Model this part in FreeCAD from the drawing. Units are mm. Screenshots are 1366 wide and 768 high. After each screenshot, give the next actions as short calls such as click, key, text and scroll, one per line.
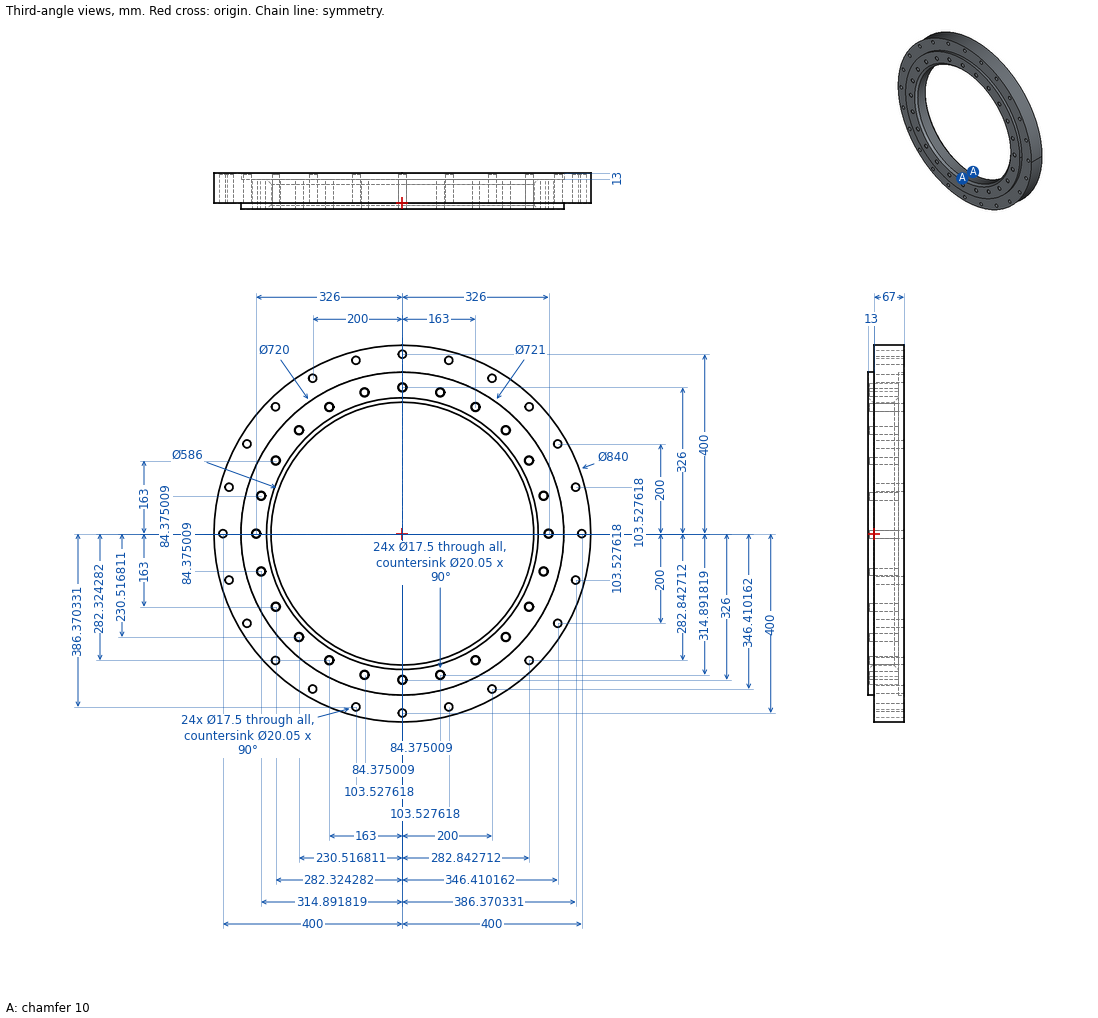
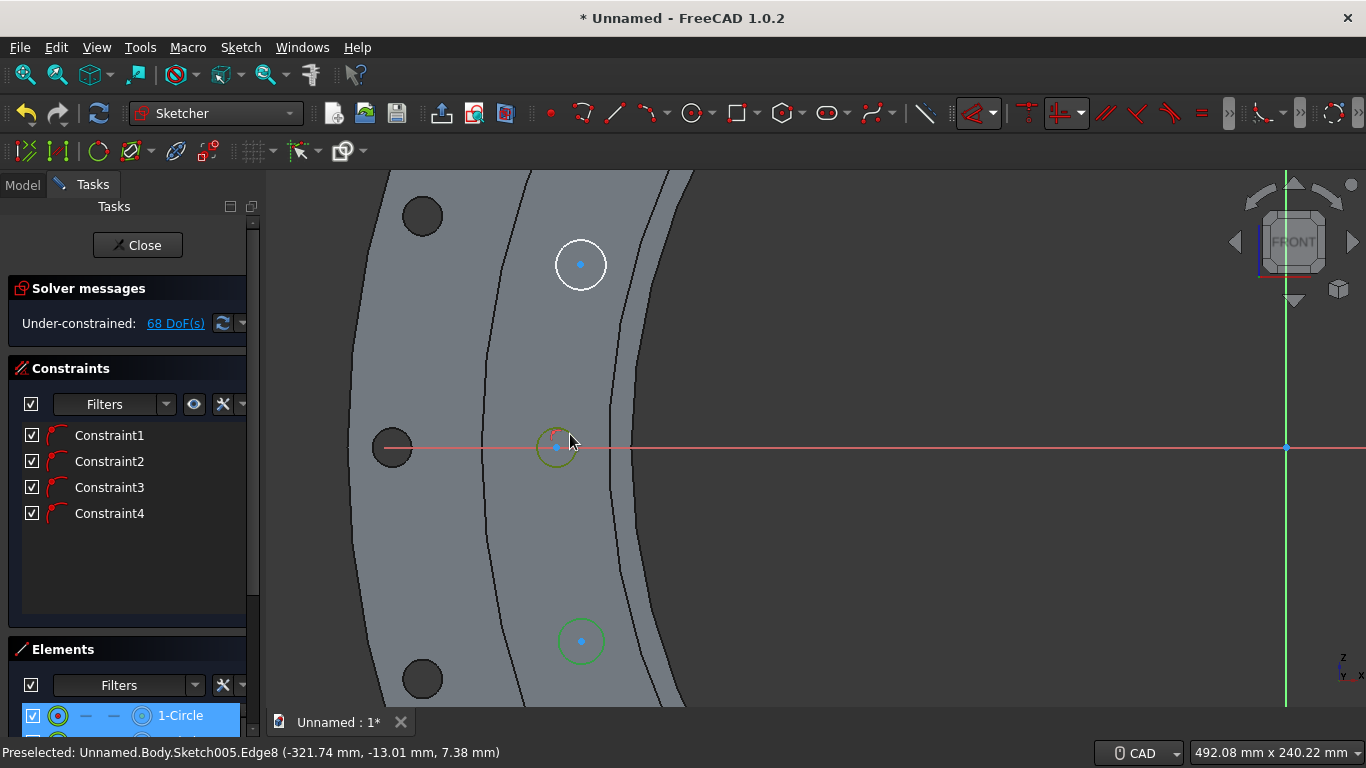
click(598, 247)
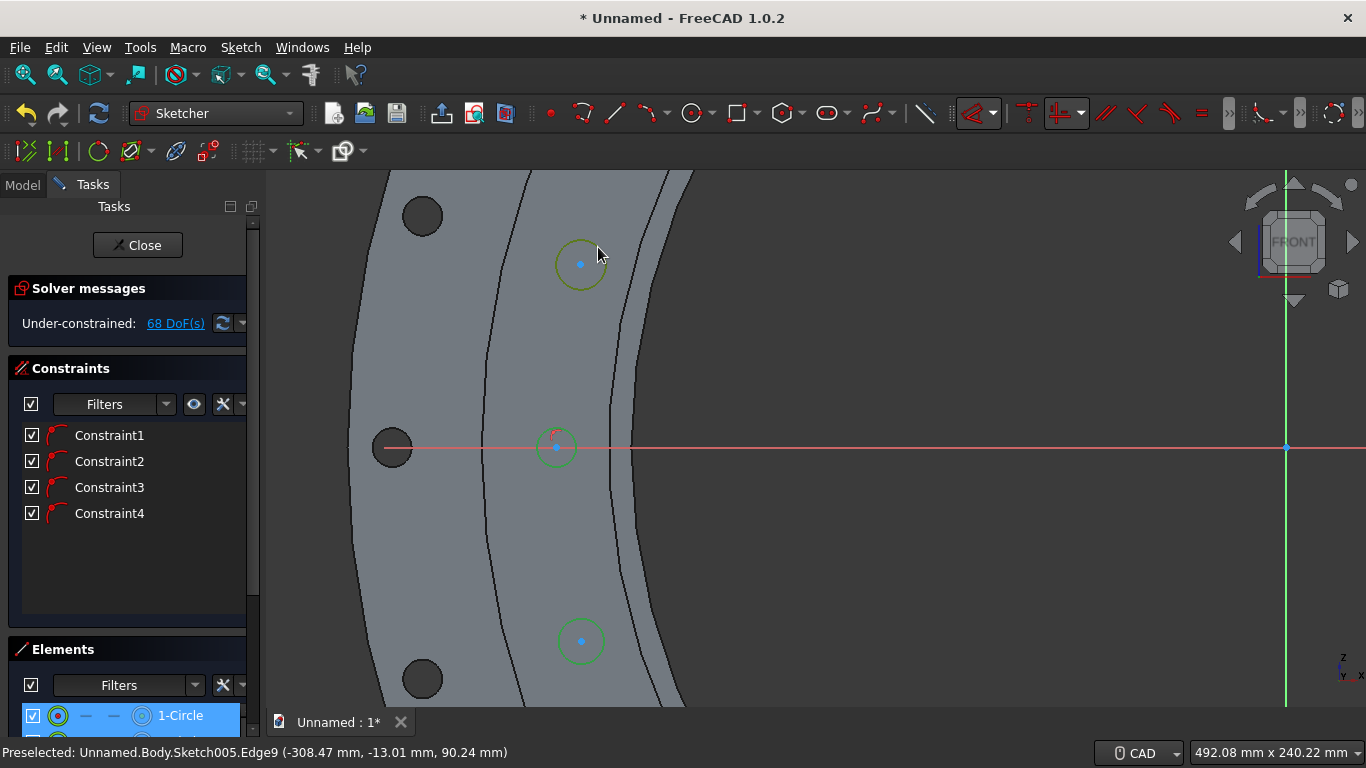
scroll(571, 436, down, 7)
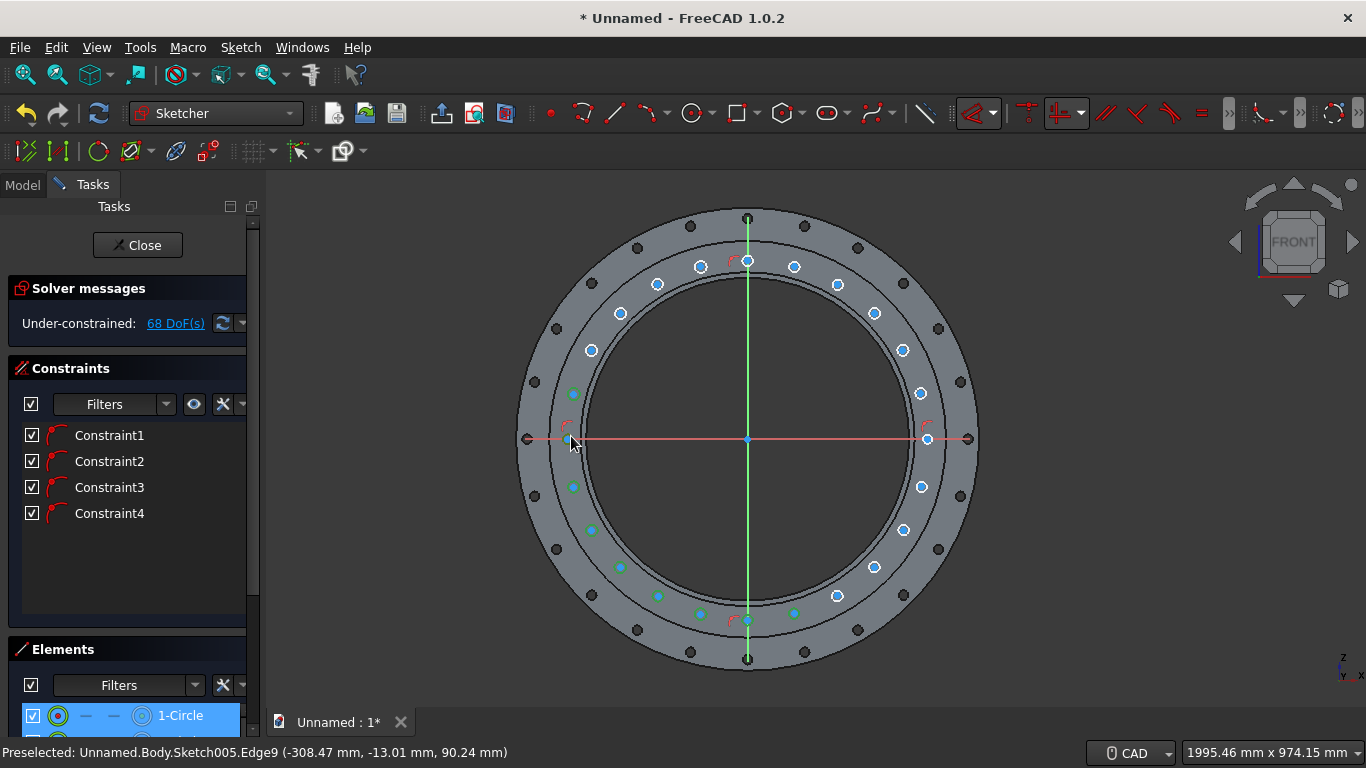
scroll(596, 347, up, 5)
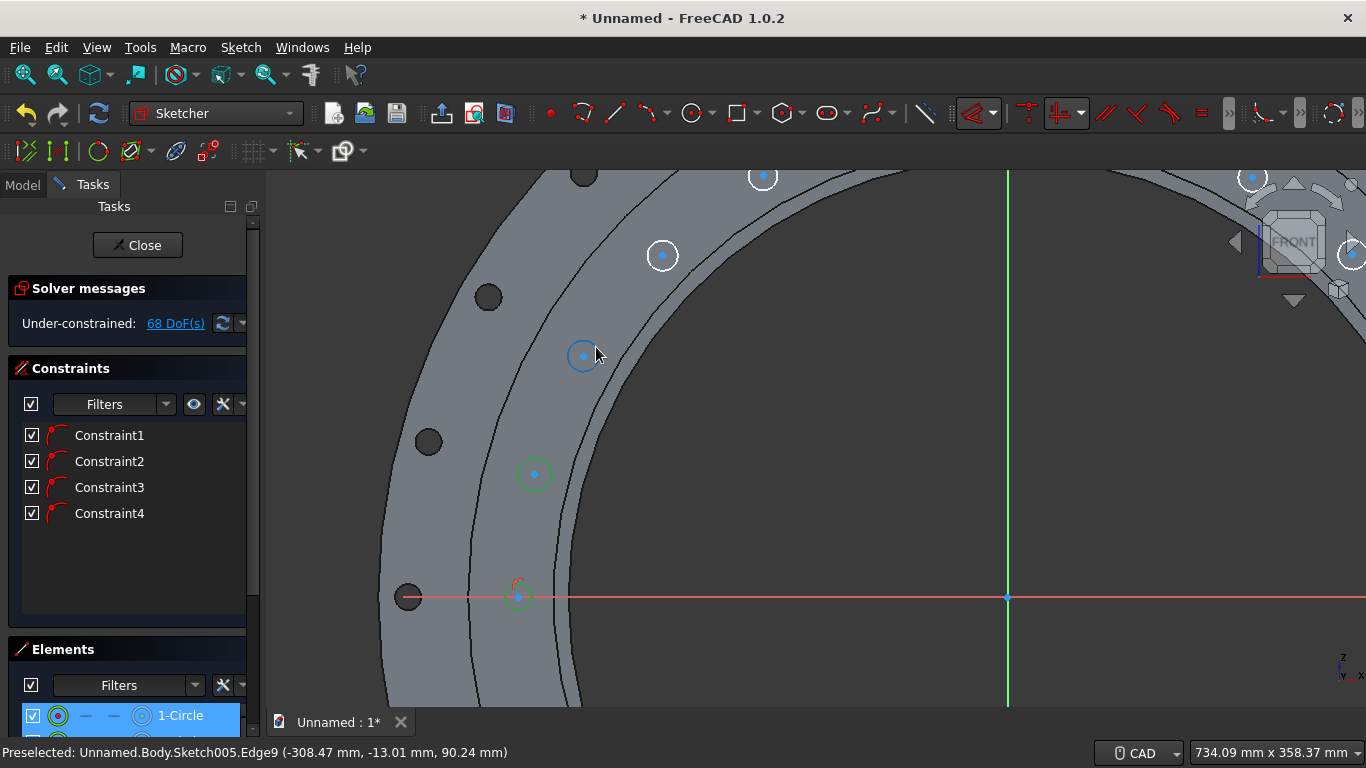
click(594, 345)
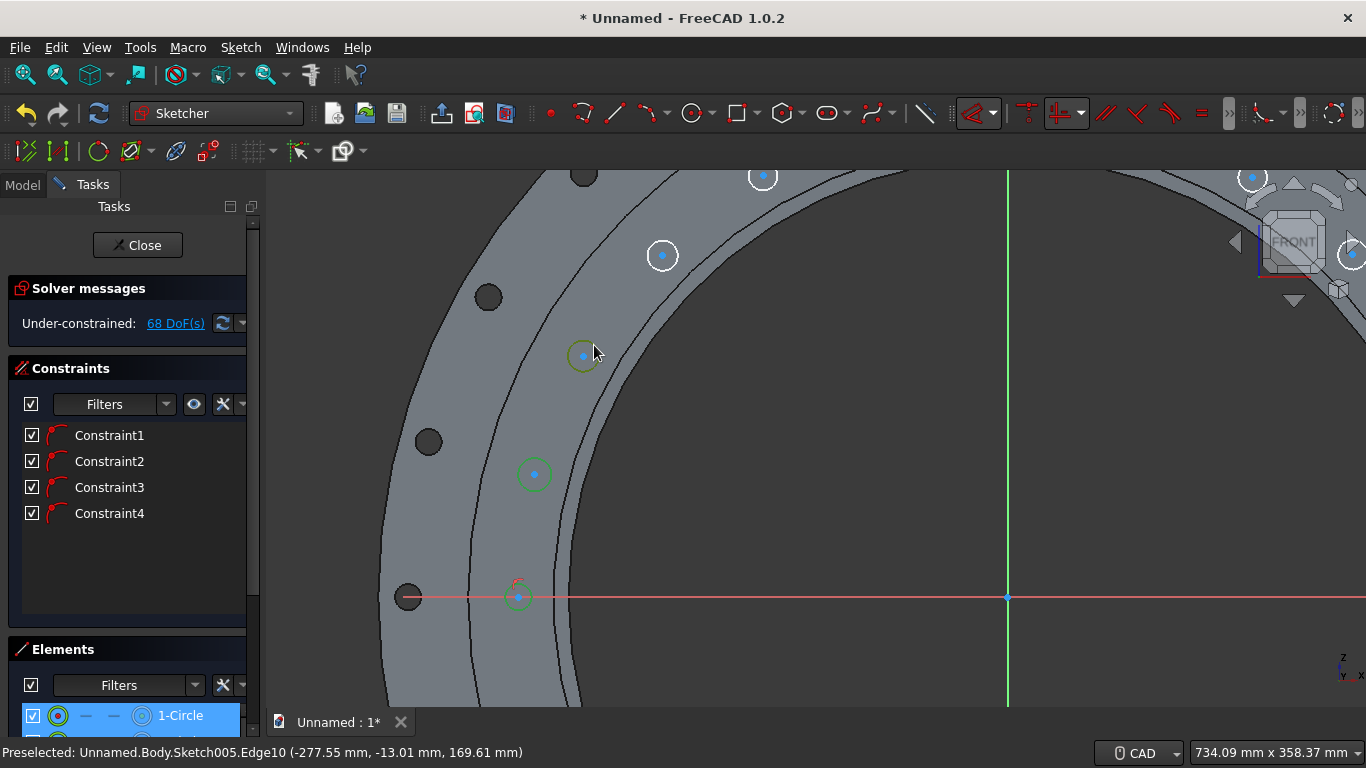
click(673, 245)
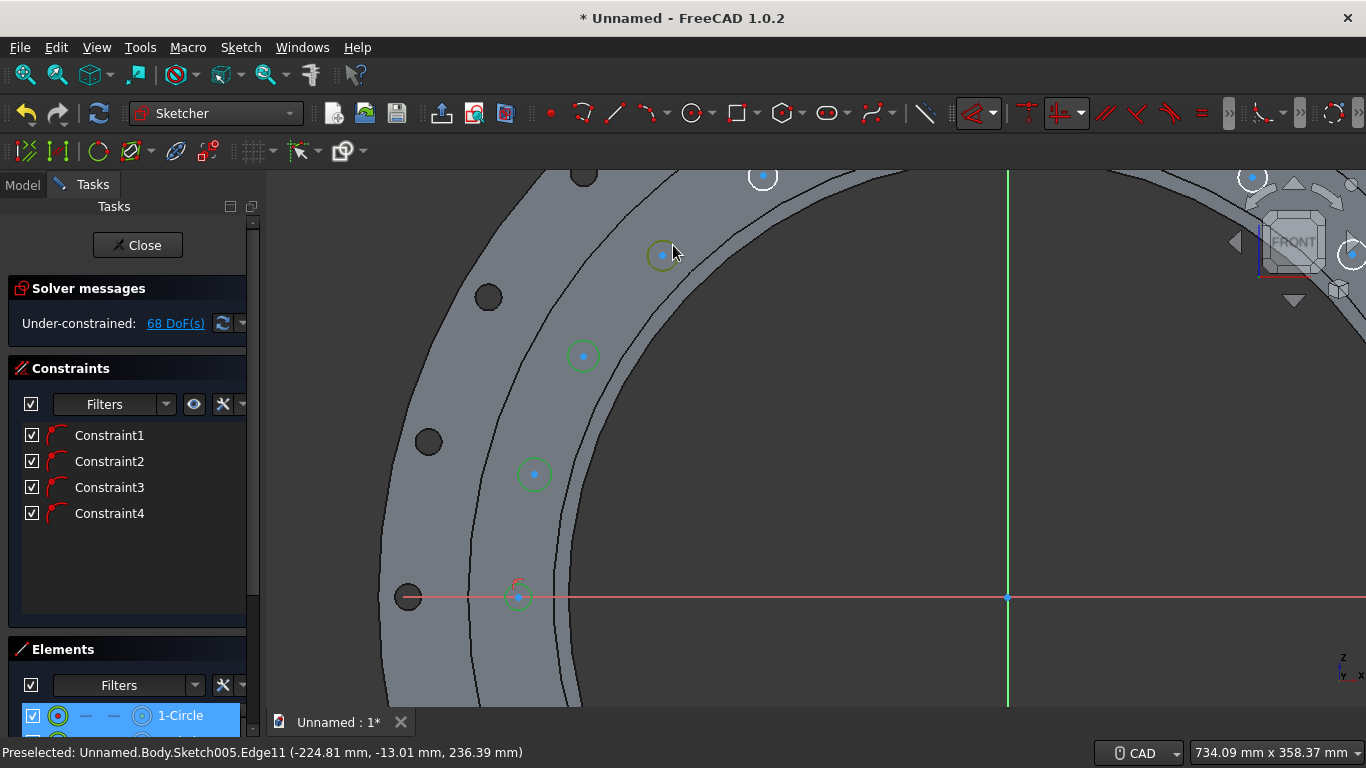
scroll(596, 346, down, 5)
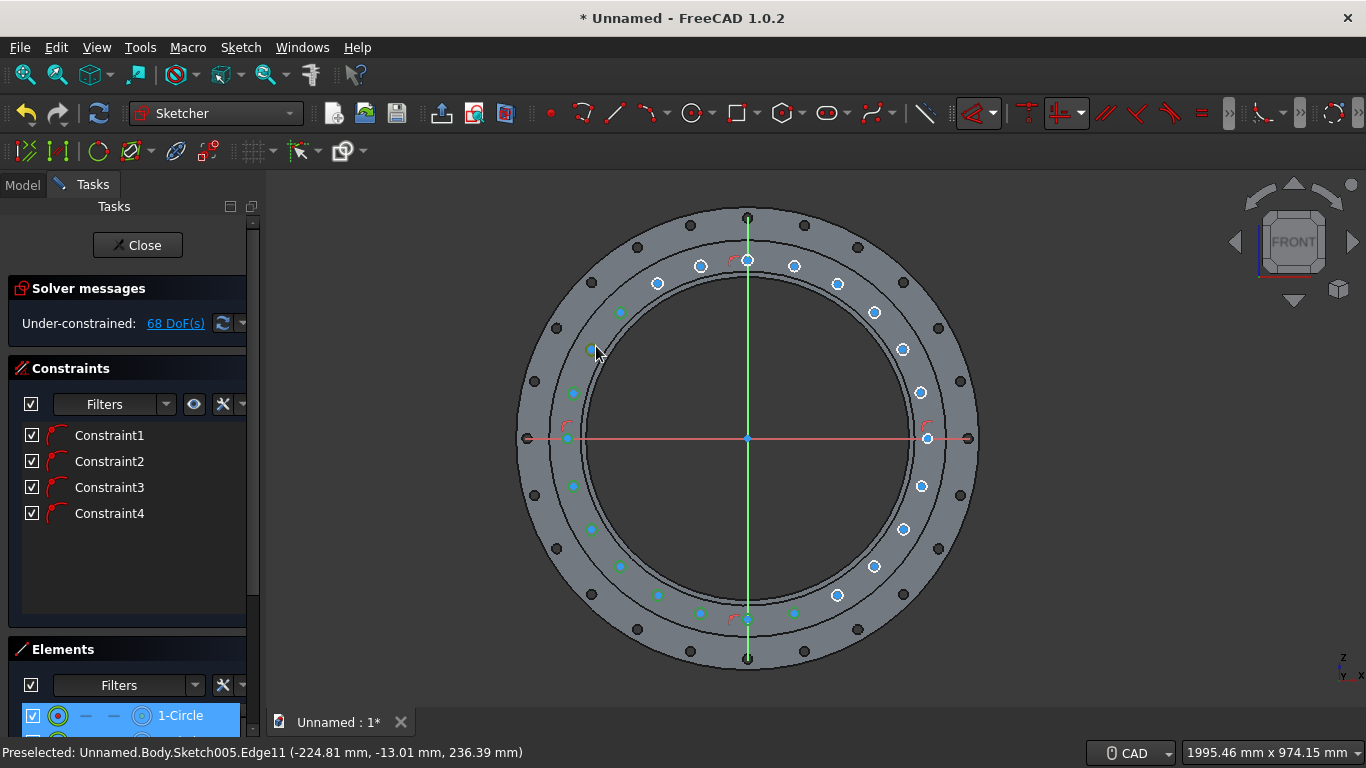
scroll(661, 280, up, 5)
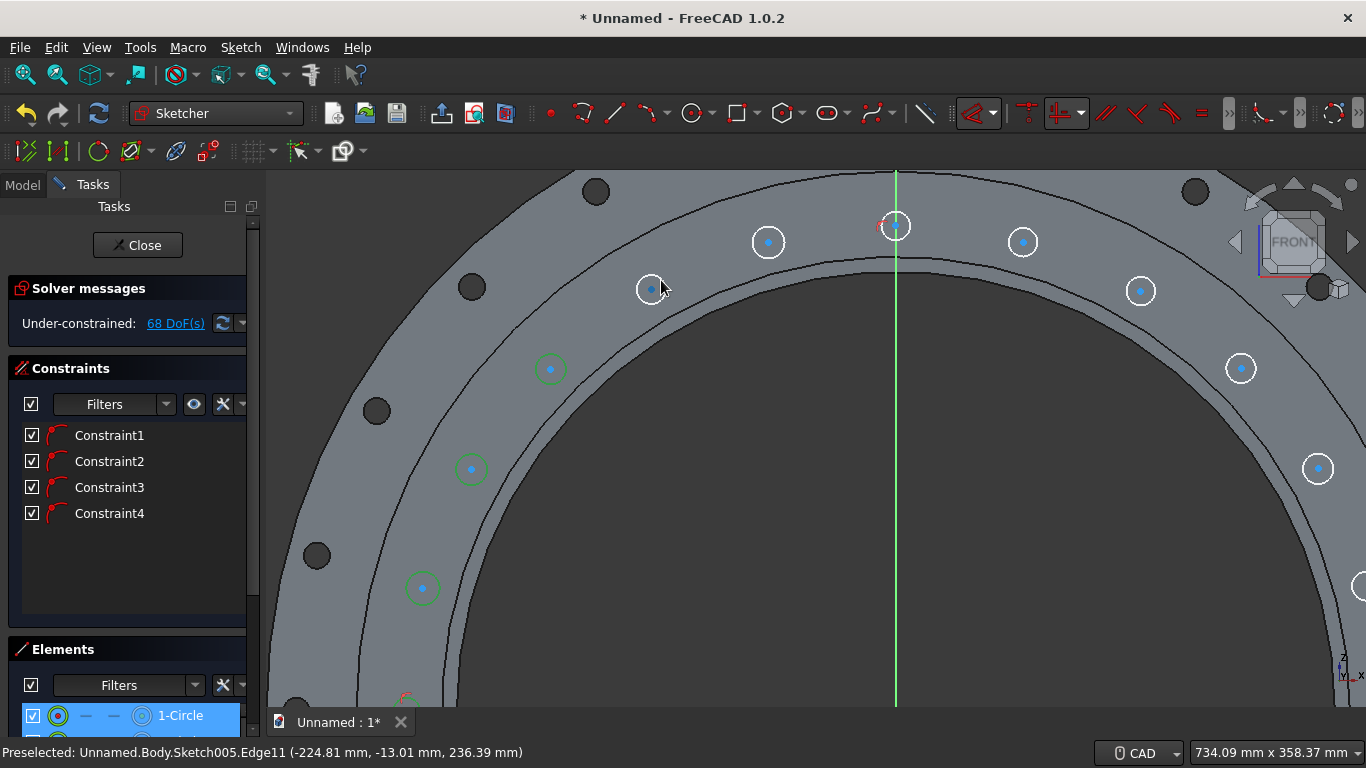
click(661, 279)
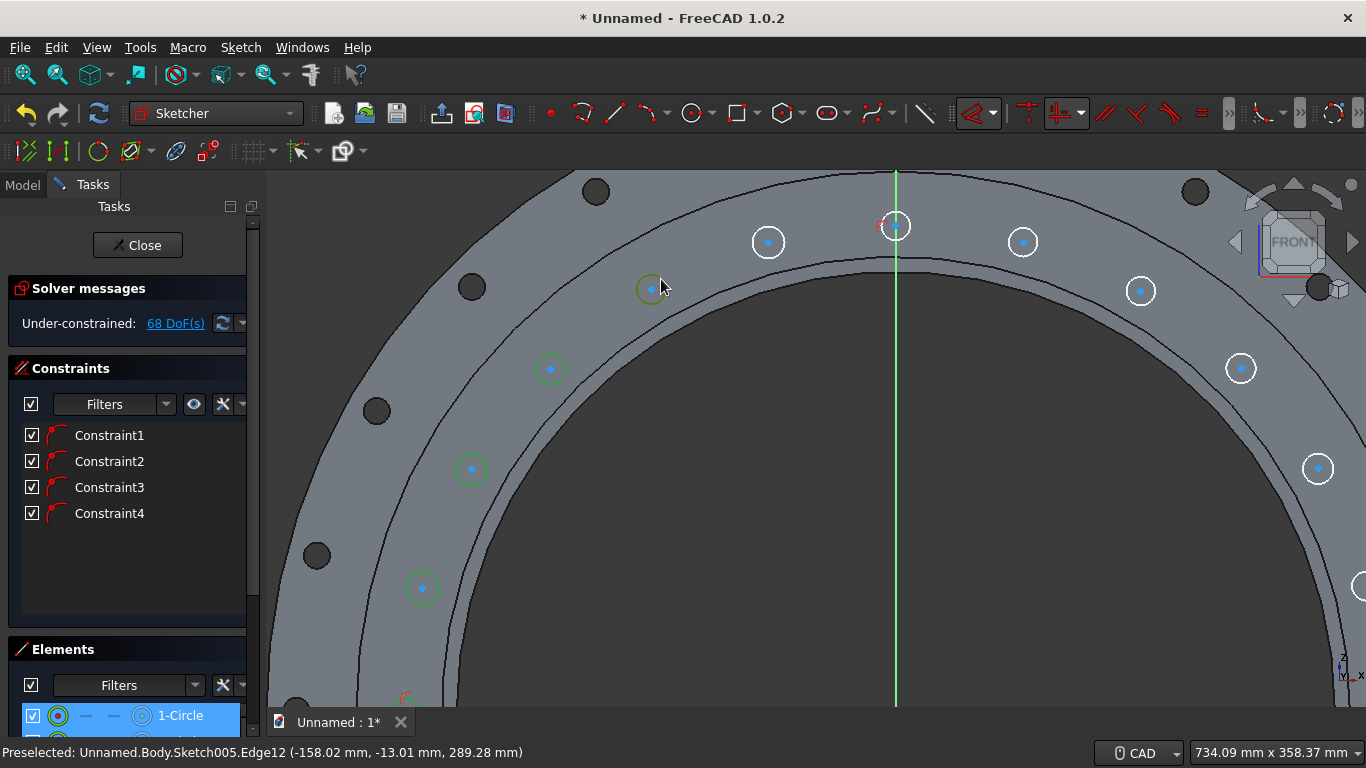
click(780, 231)